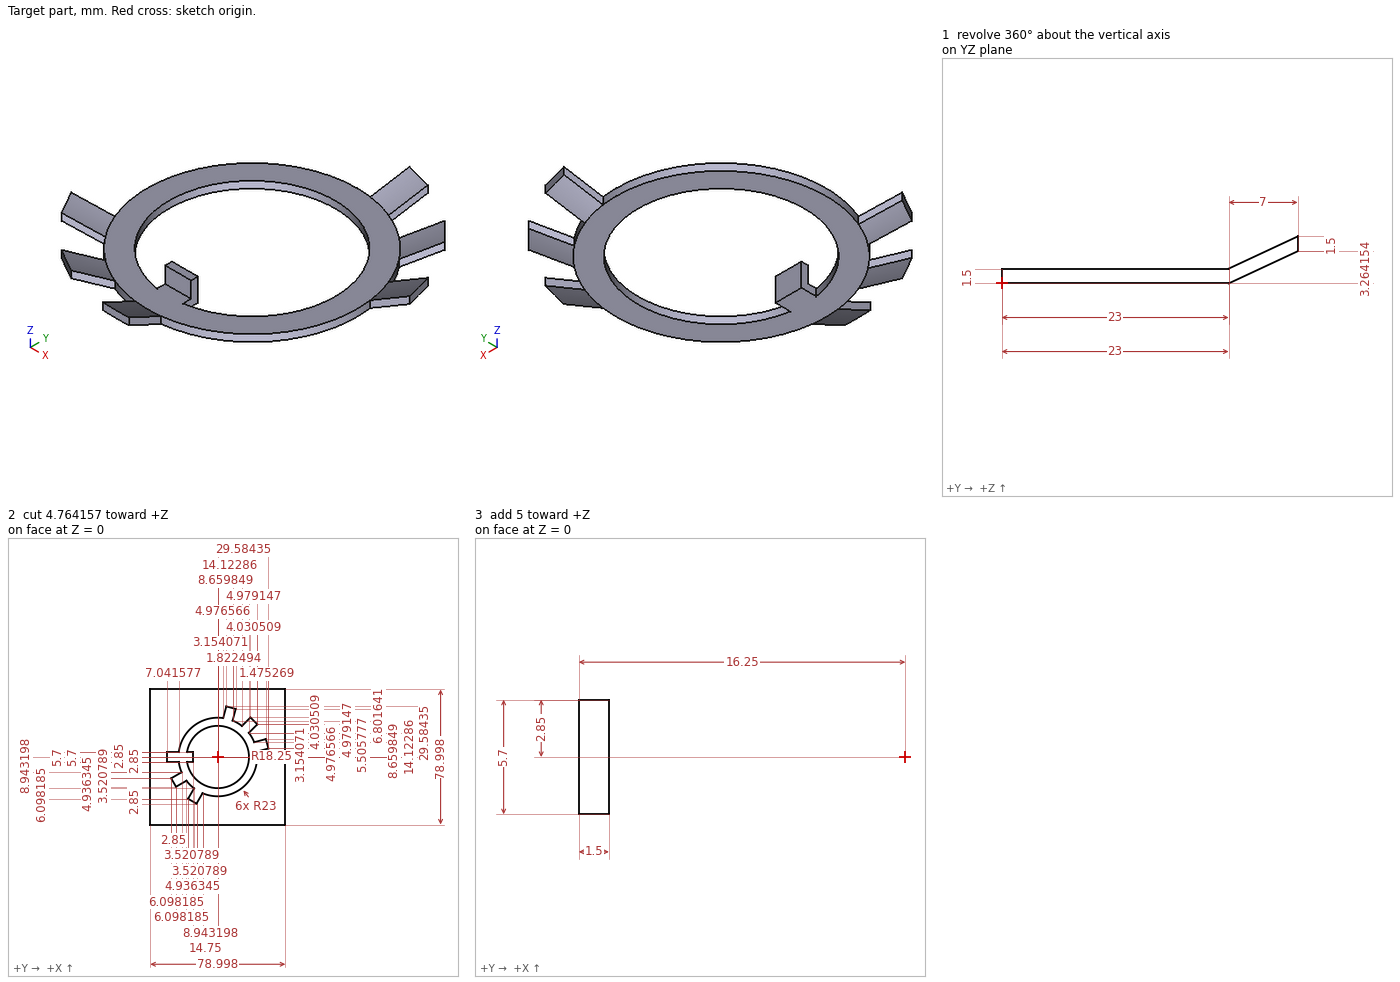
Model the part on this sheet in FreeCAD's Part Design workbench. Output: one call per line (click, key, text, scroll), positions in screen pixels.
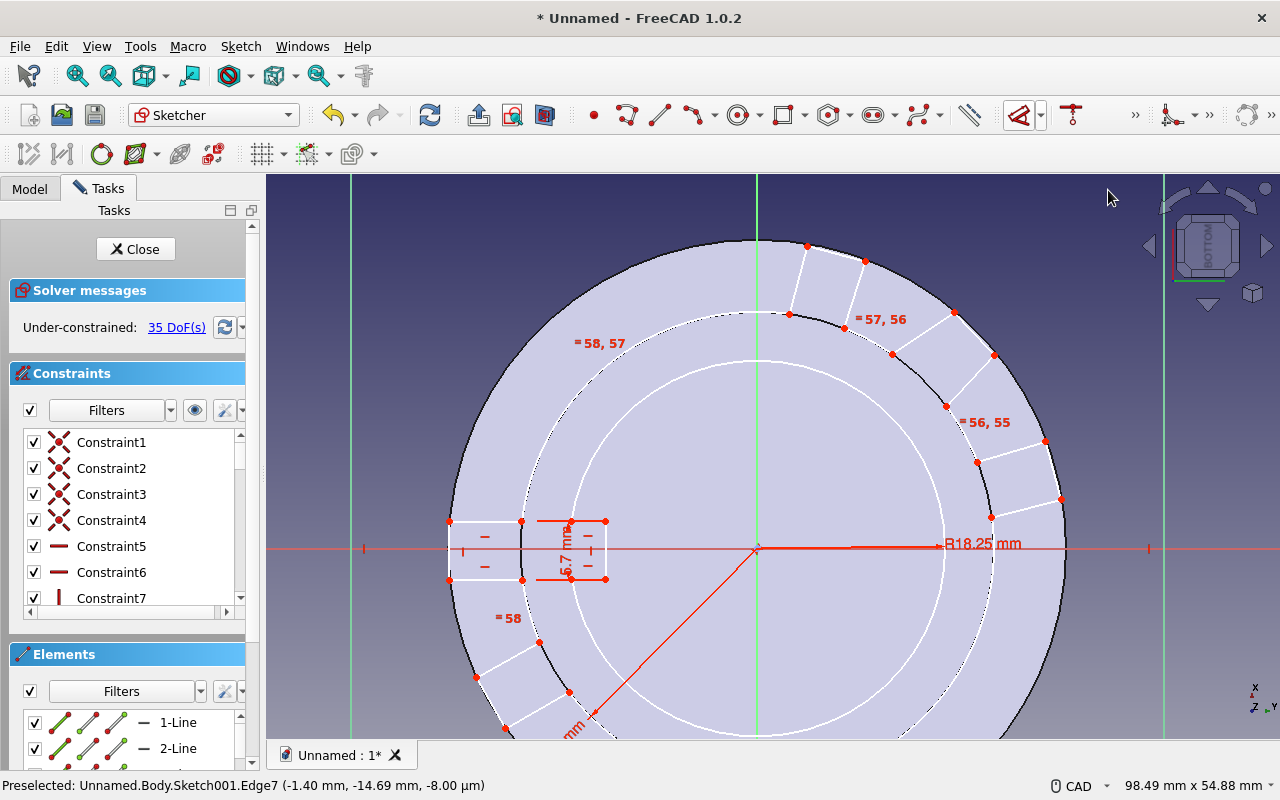
scroll(449, 540, up, 3)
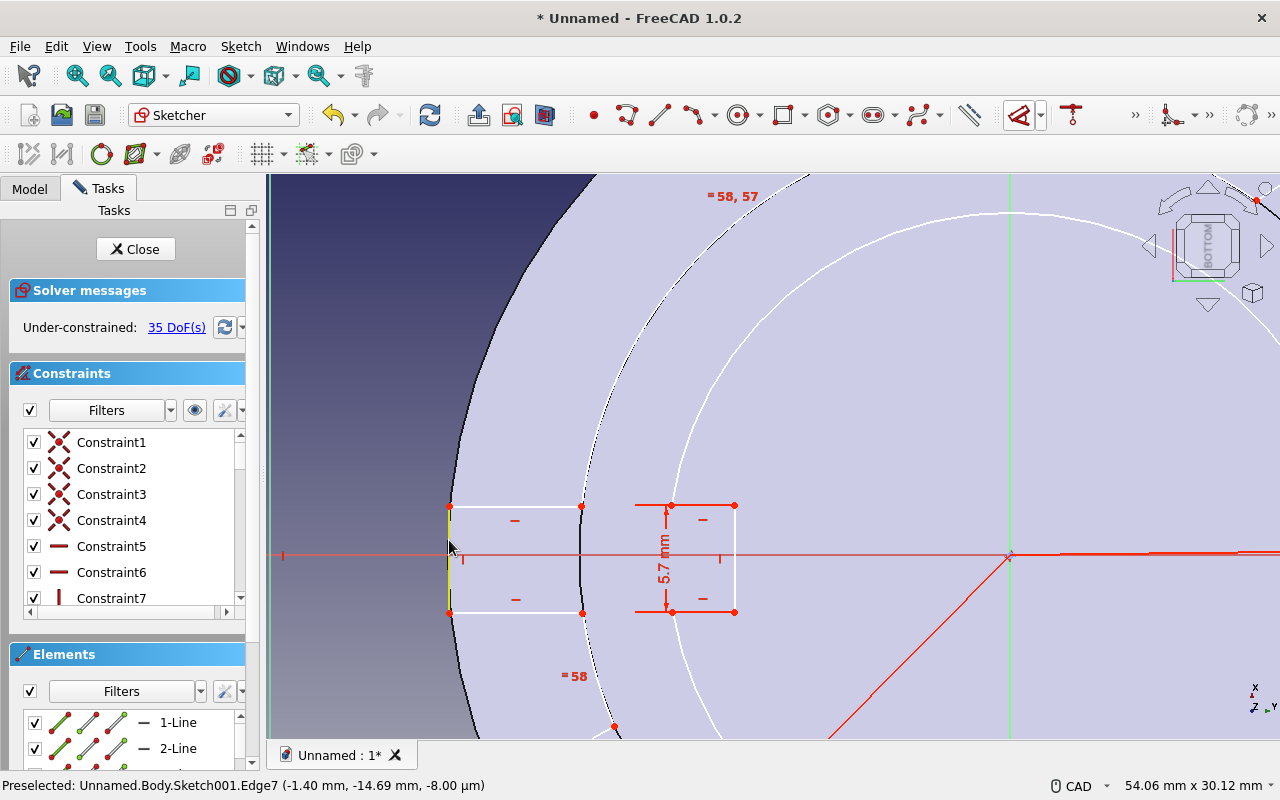
click(449, 539)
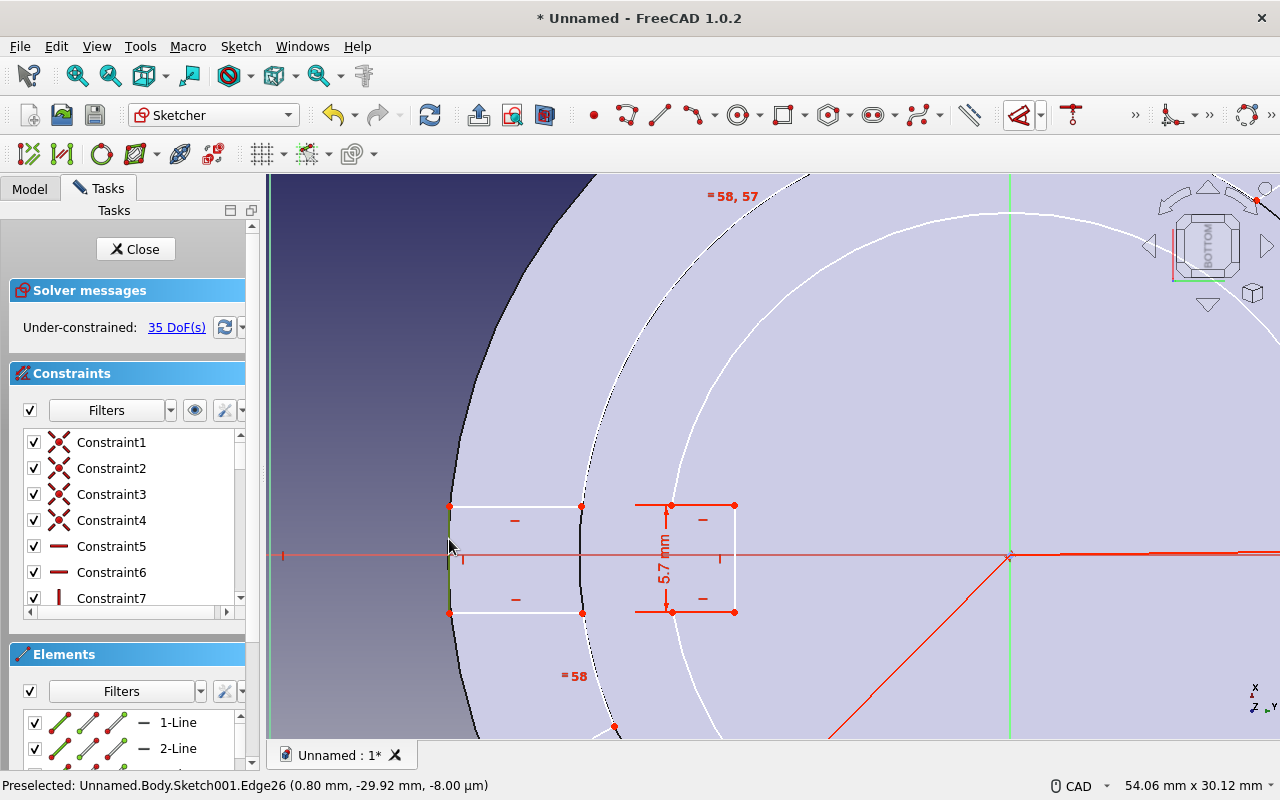
click(1040, 116)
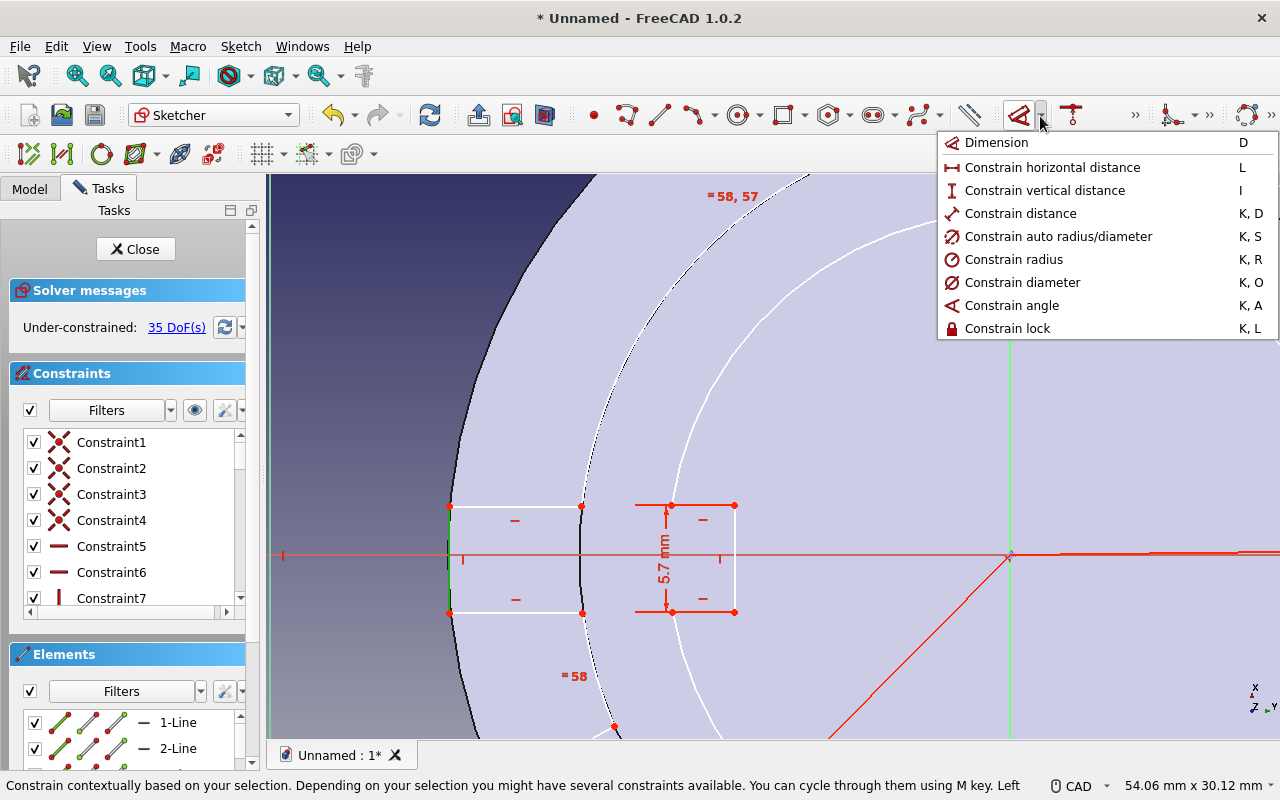
click(1108, 190)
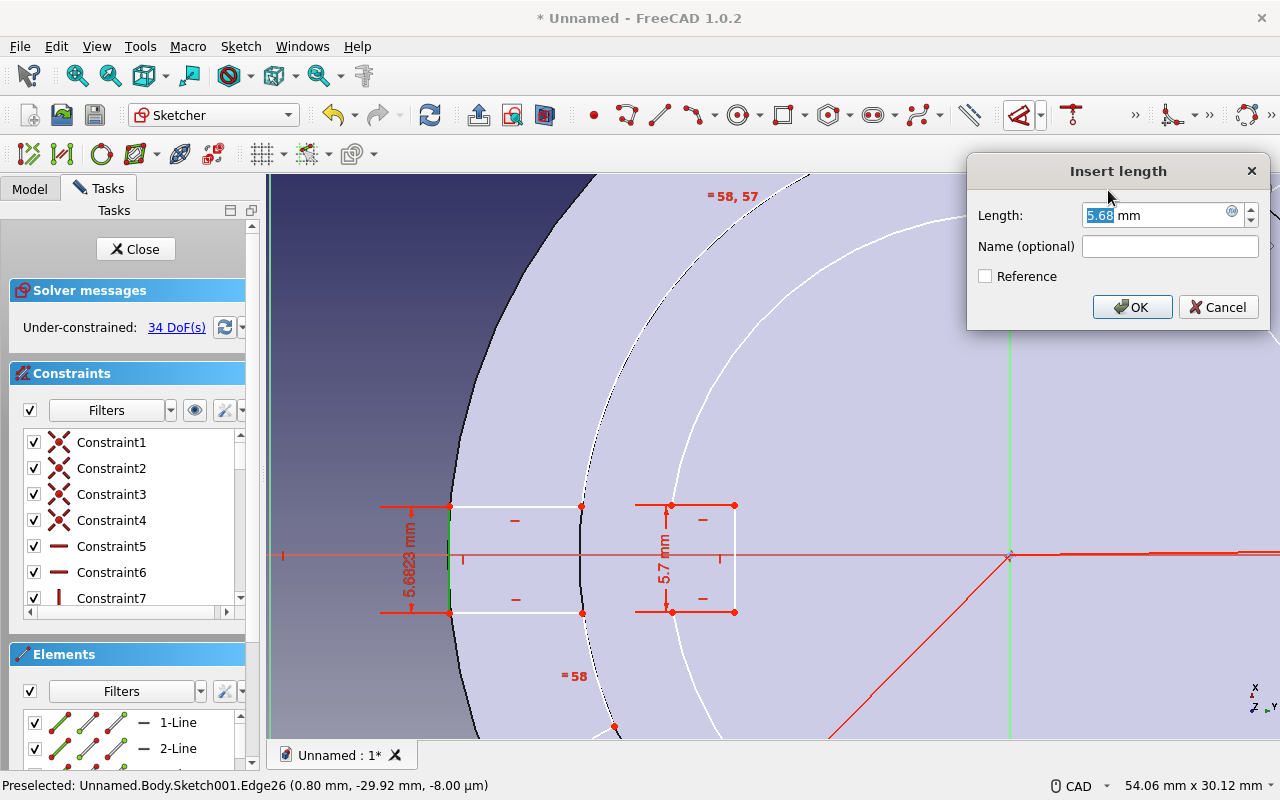
text(5.7)
key(Return)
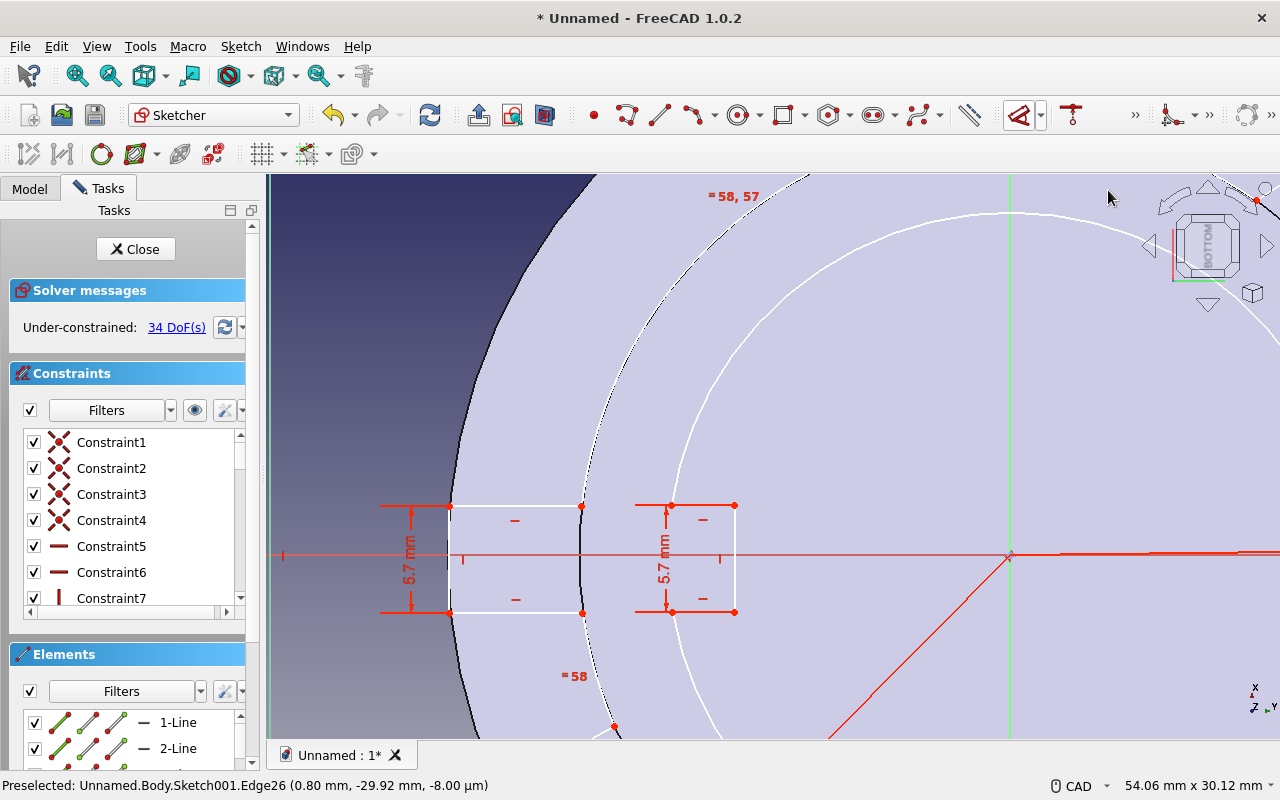
click(673, 612)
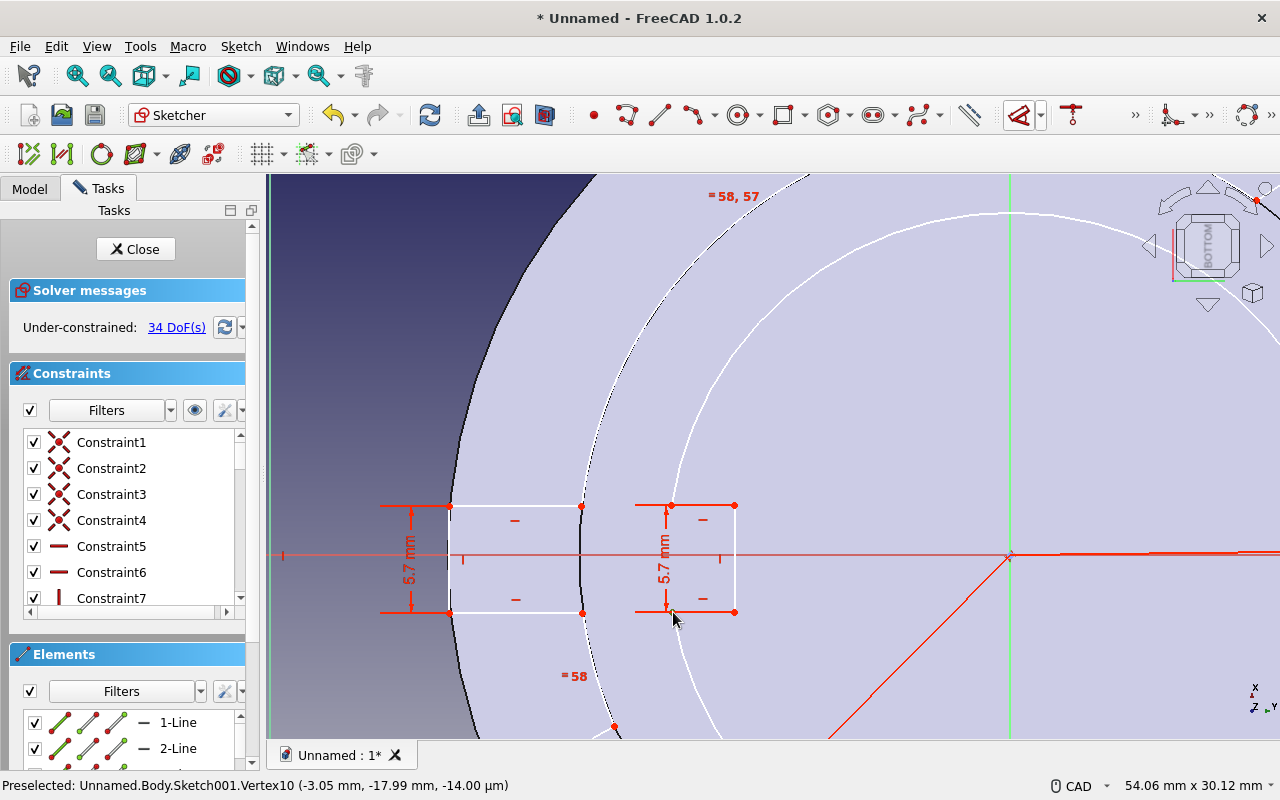
click(1040, 116)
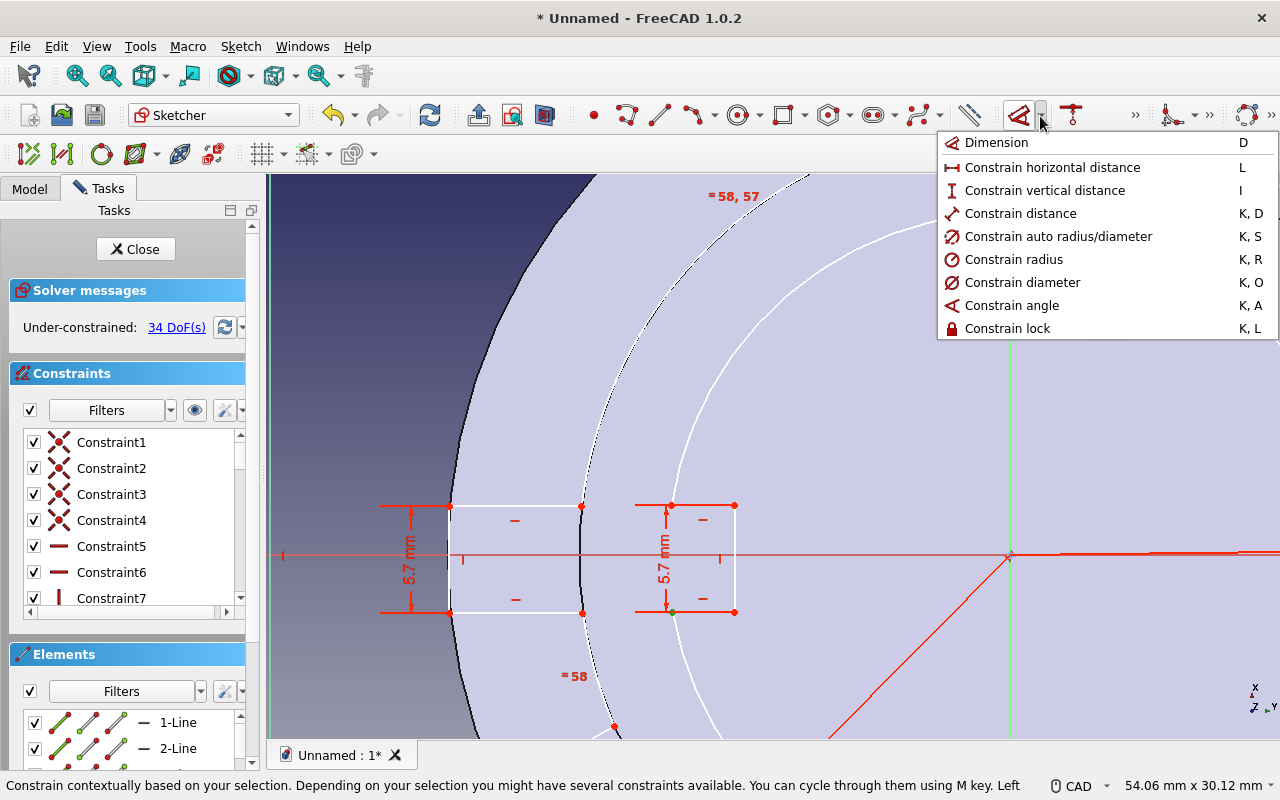
click(1108, 190)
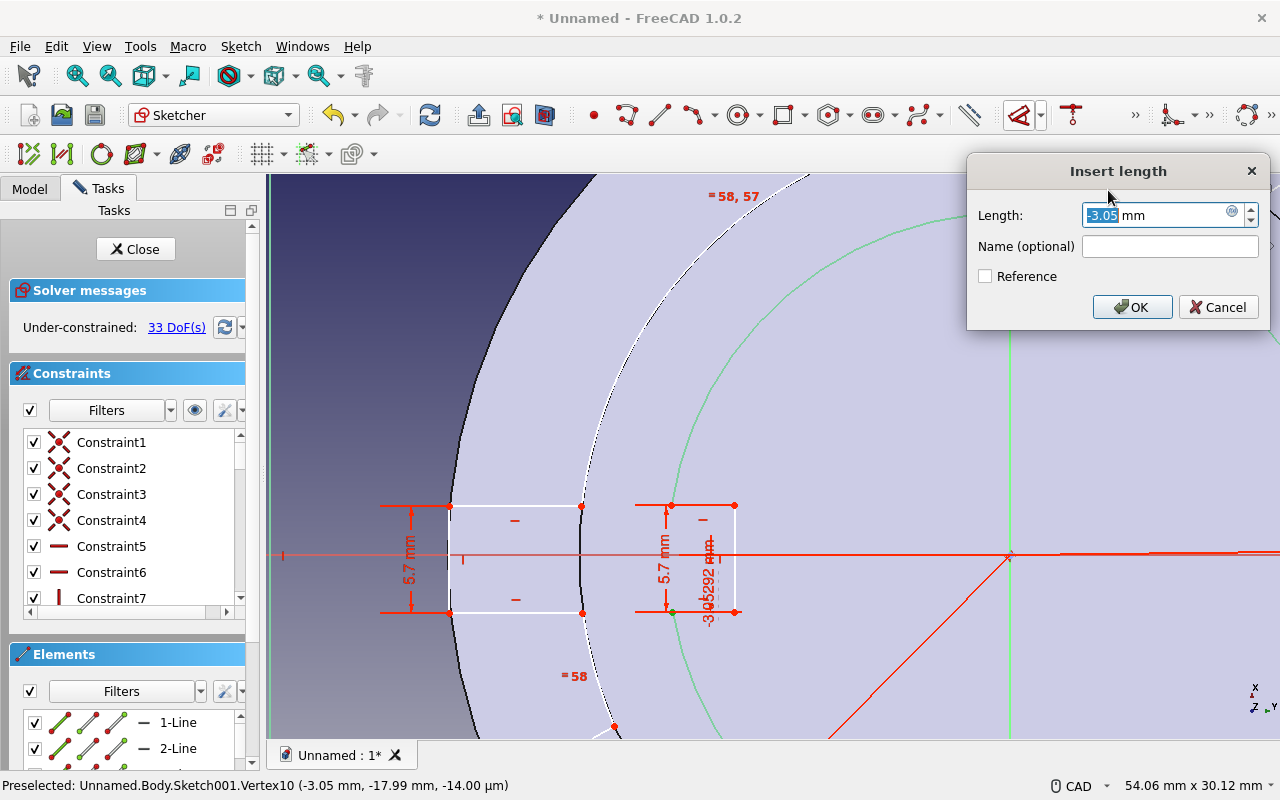
text(-2.85)
key(Return)